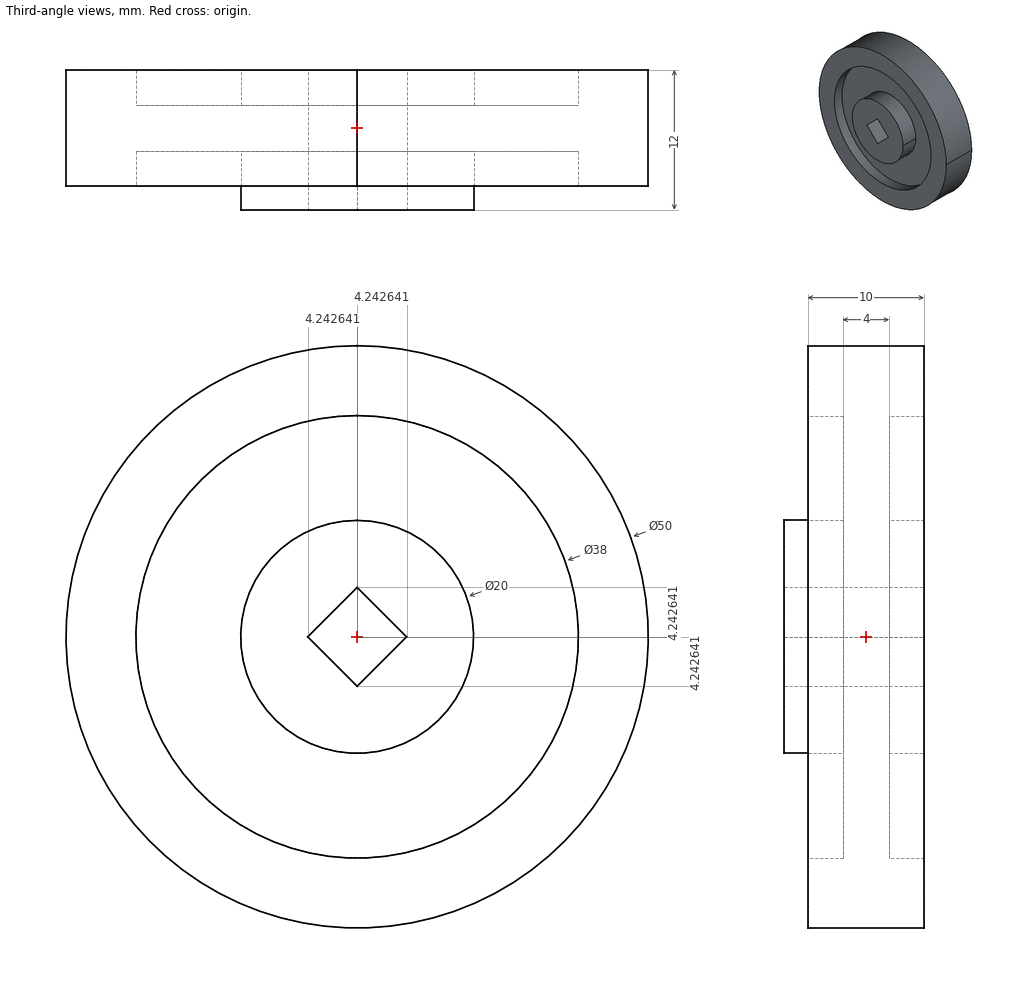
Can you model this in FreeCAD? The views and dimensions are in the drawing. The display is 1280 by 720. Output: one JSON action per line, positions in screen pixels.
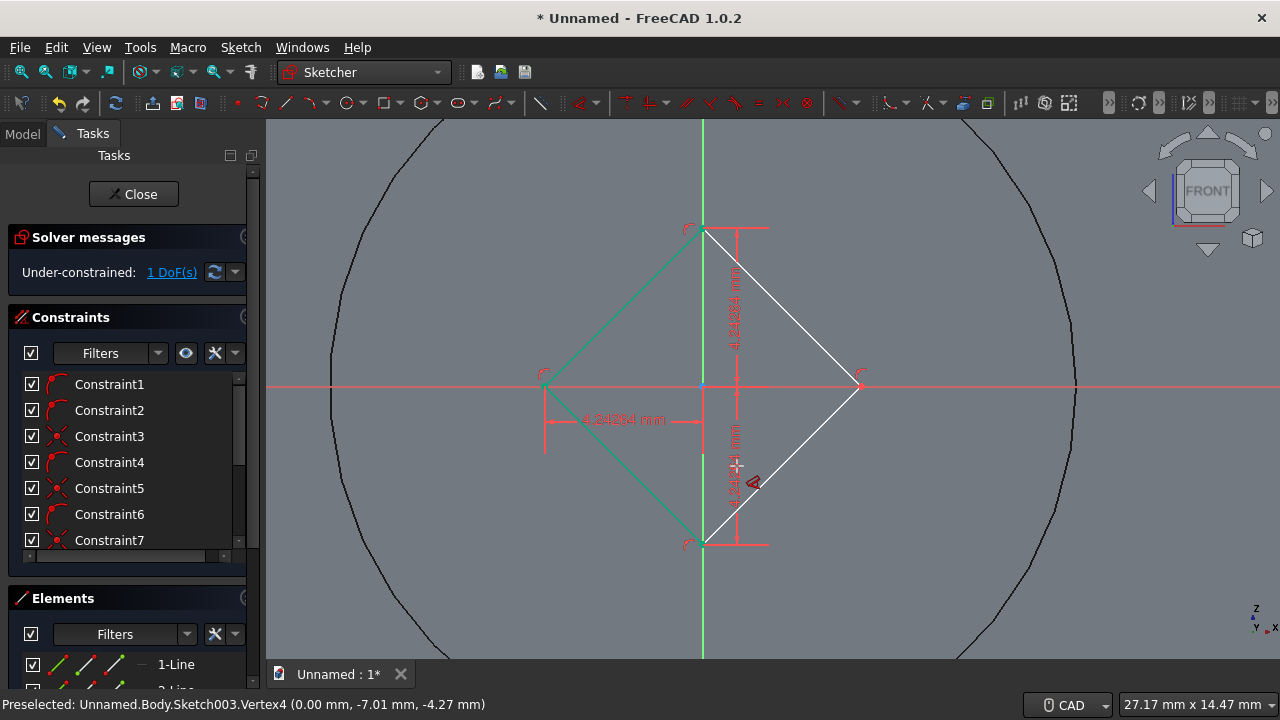
{"action": "left_click", "coordinate": [861, 387]}
{"action": "left_click", "coordinate": [782, 421]}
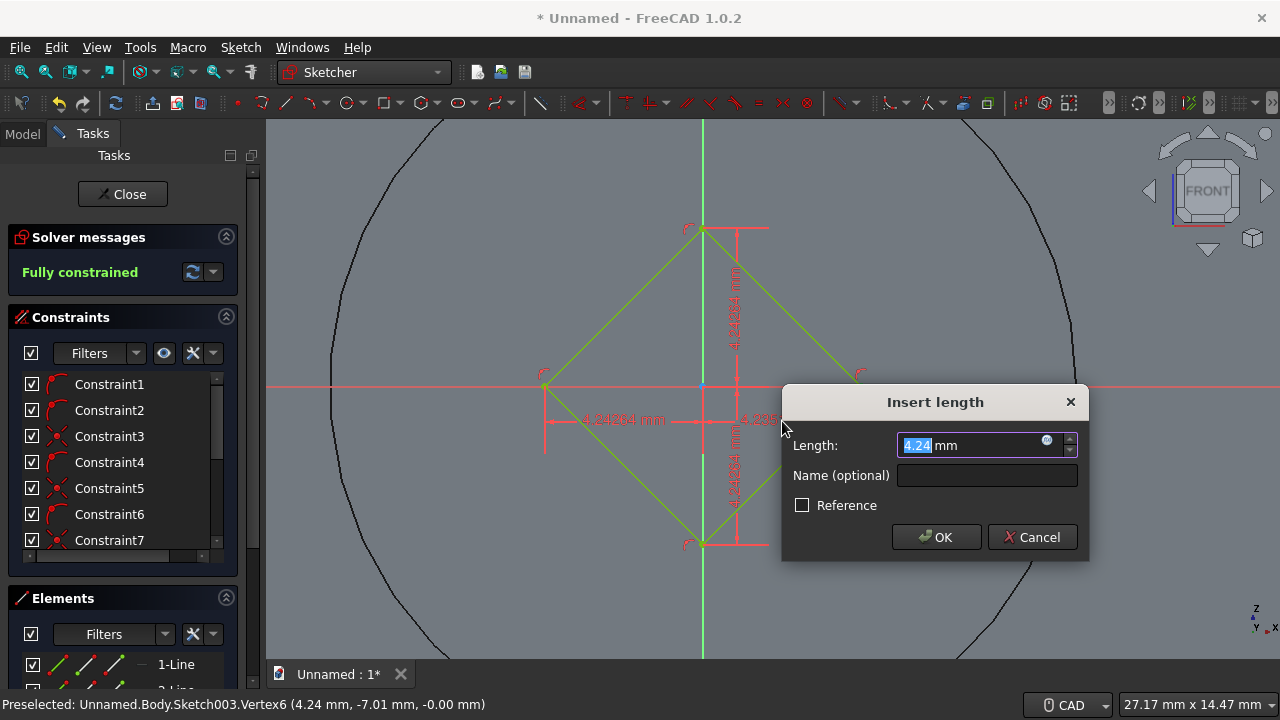
{"action": "type", "text": "4.242641"}
{"action": "key", "text": "Return"}
{"action": "key", "text": "Escape"}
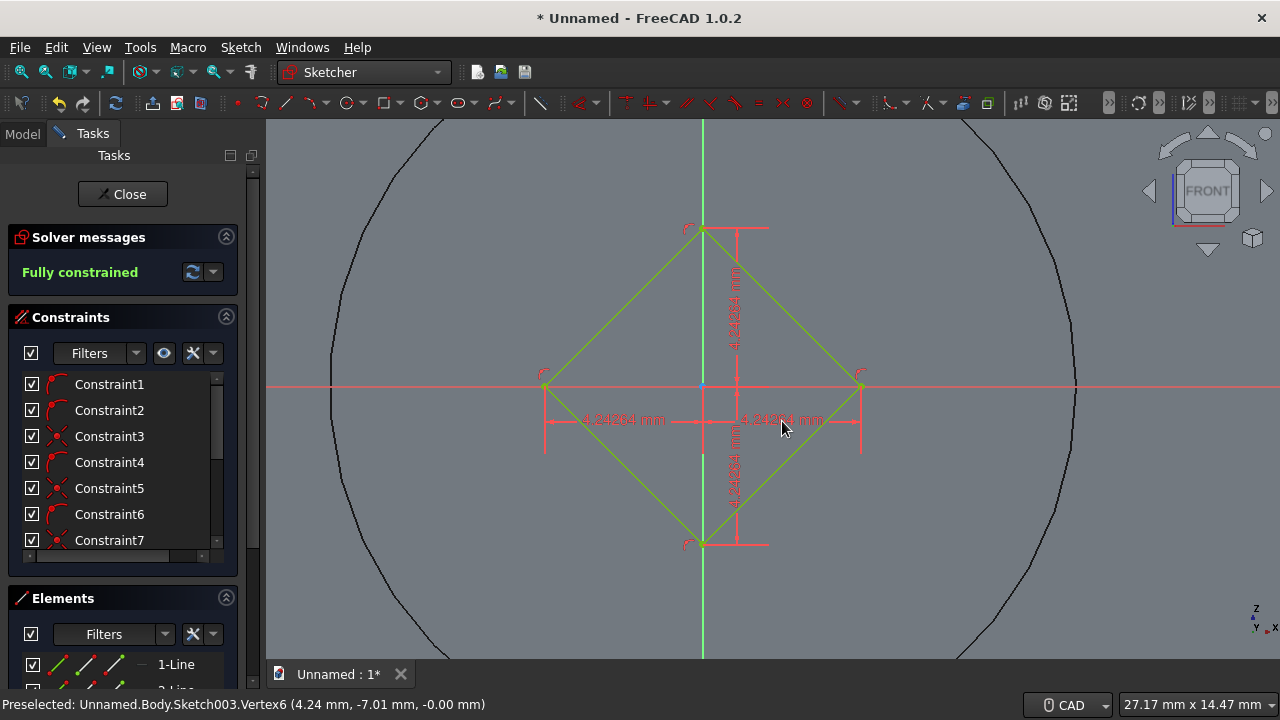
{"action": "left_click", "coordinate": [123, 194]}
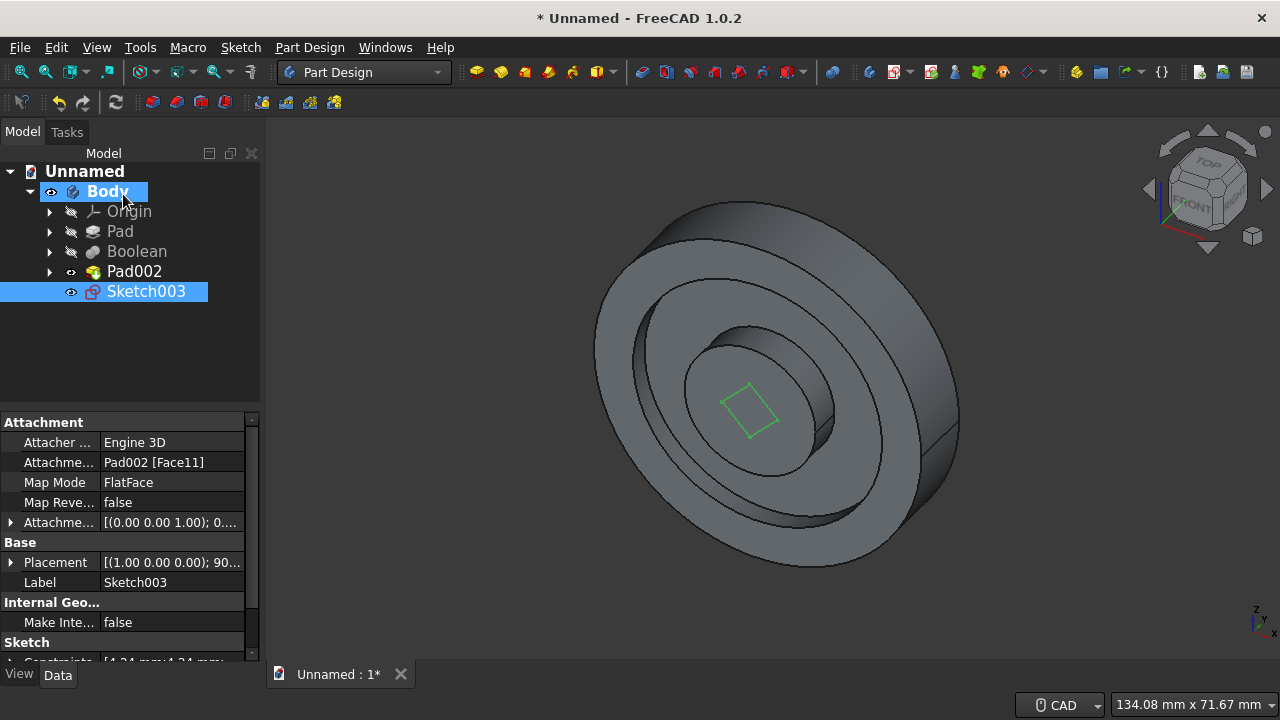
{"action": "left_click", "coordinate": [644, 72]}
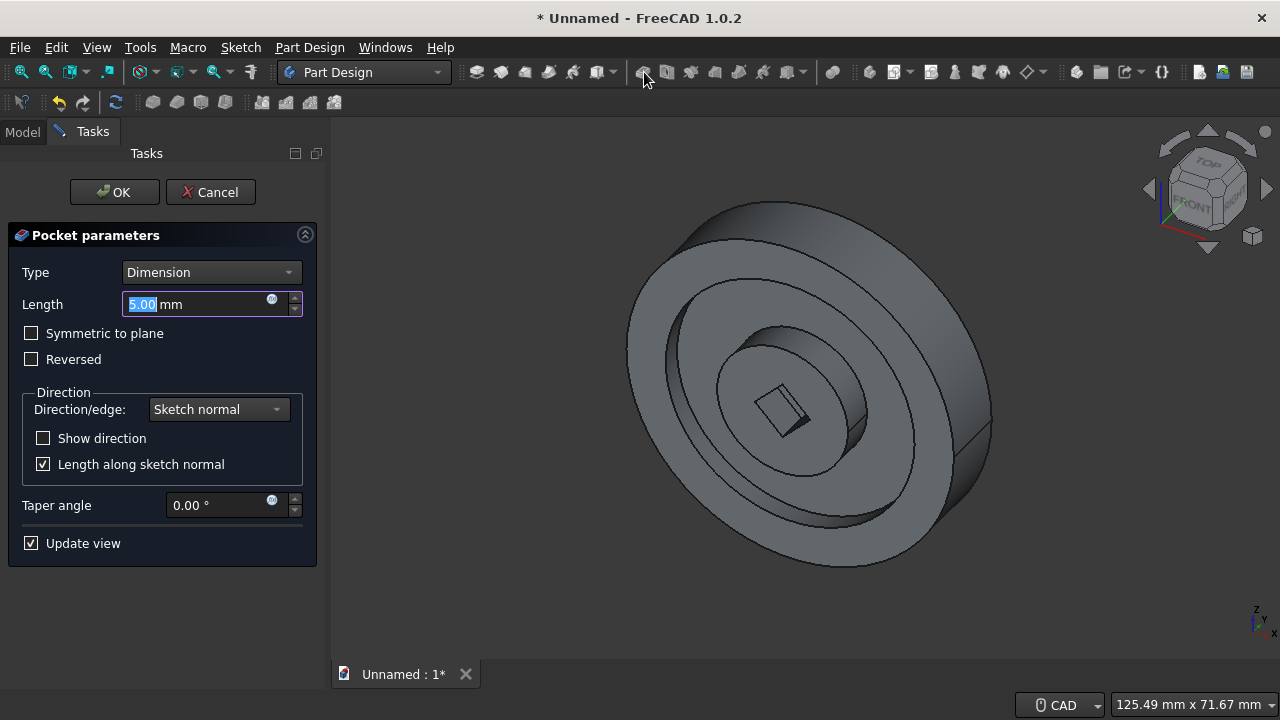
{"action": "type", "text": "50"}
{"action": "key", "text": "Tab"}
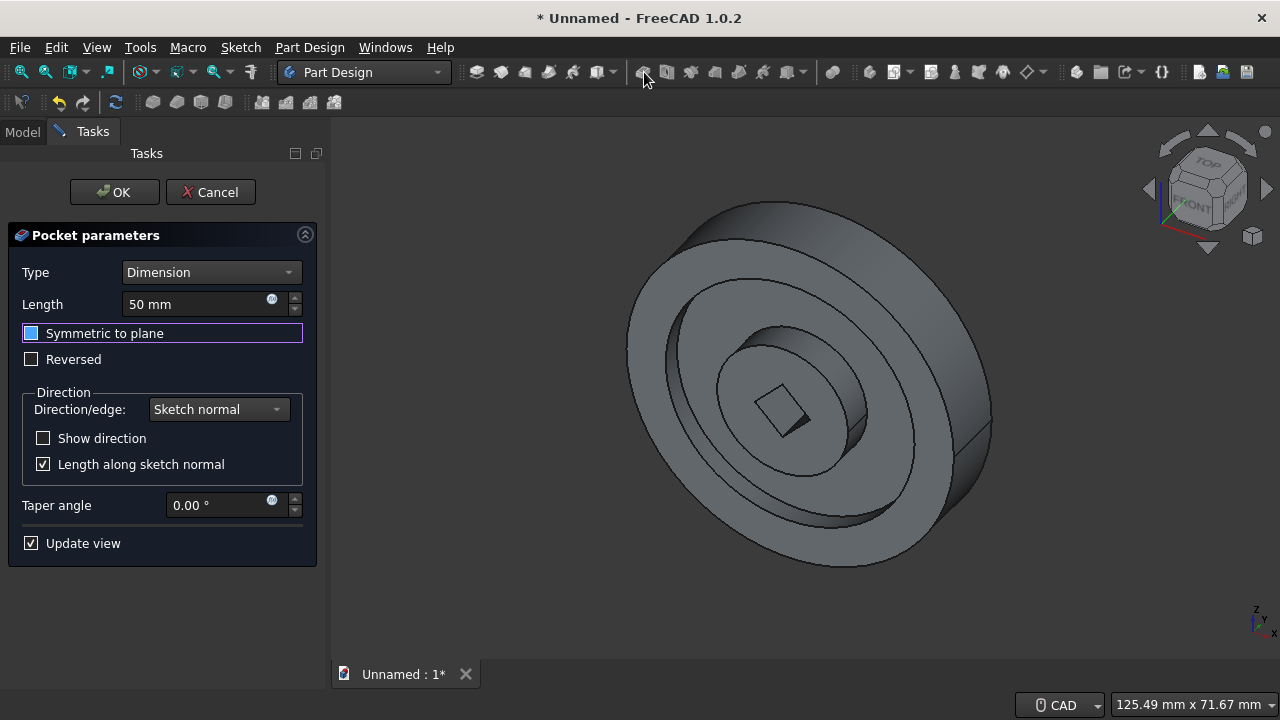
{"action": "left_click", "coordinate": [115, 192]}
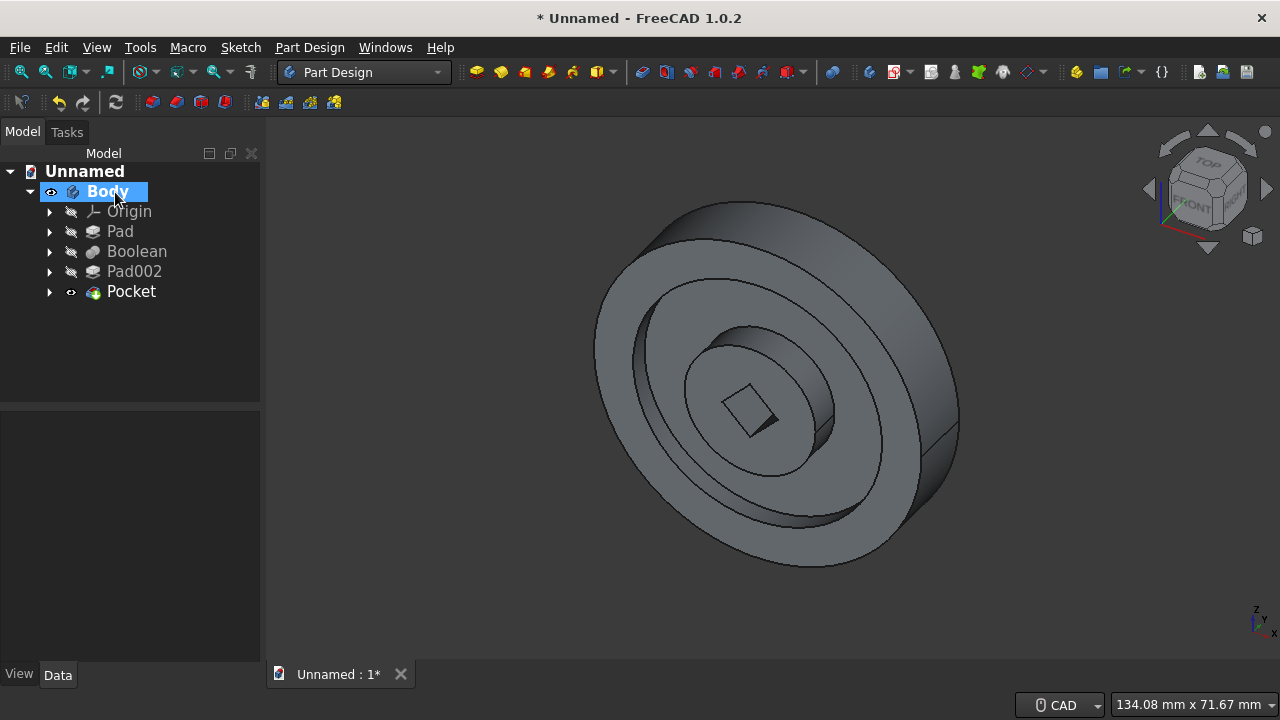
{"action": "key", "text": "0"}